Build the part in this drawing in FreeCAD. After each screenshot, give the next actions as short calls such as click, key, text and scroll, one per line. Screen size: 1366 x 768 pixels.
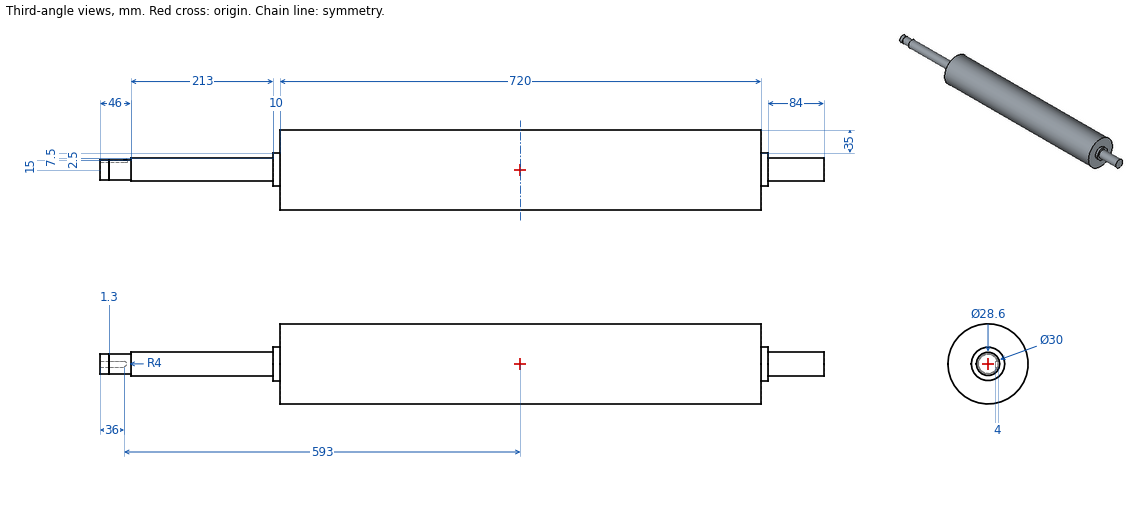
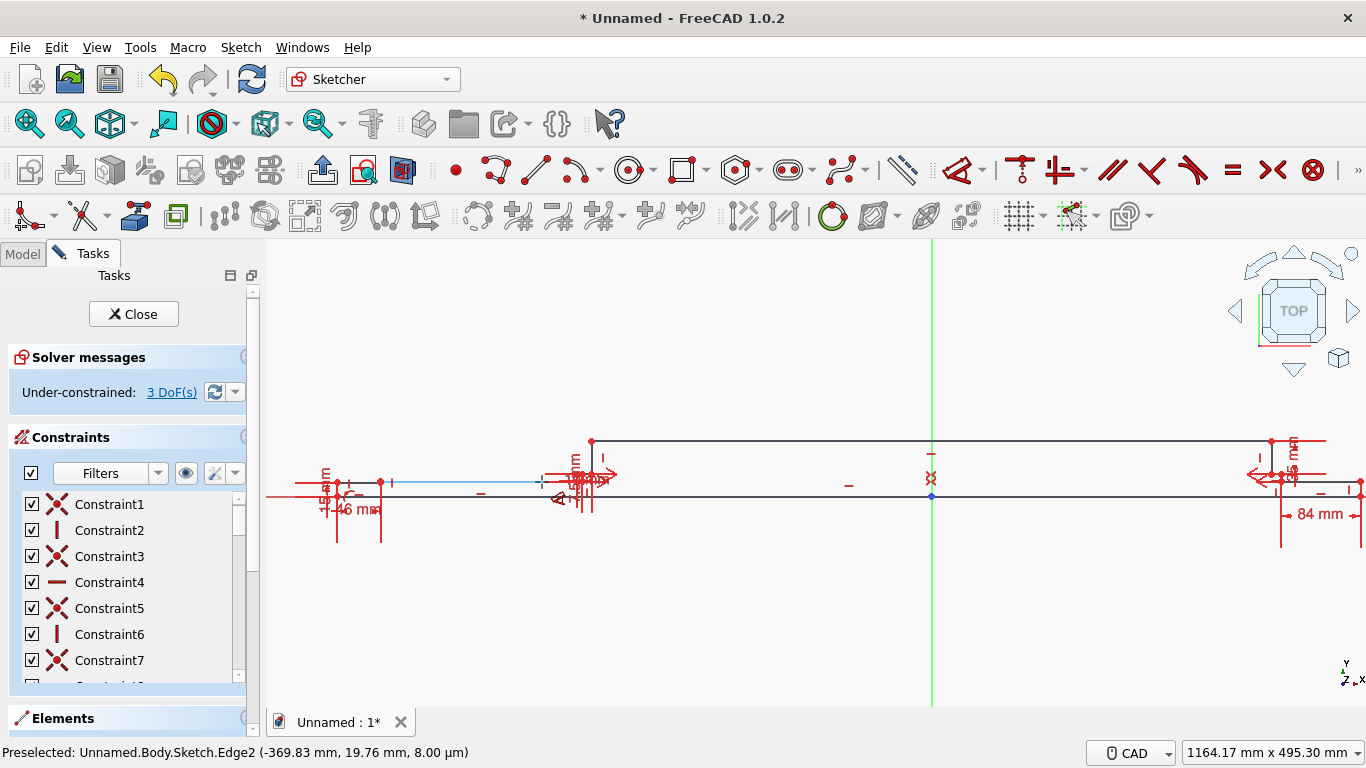
click(542, 481)
click(482, 515)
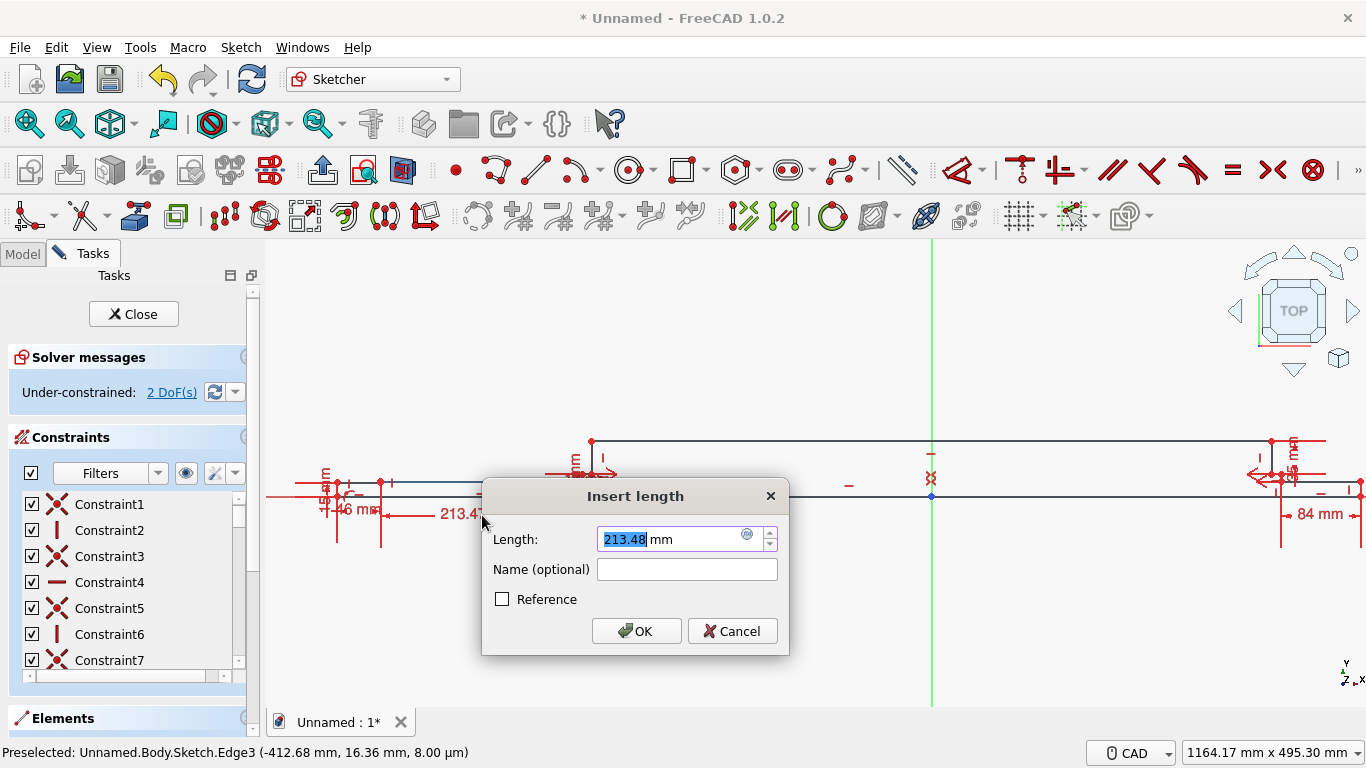
text(213)
key(Return)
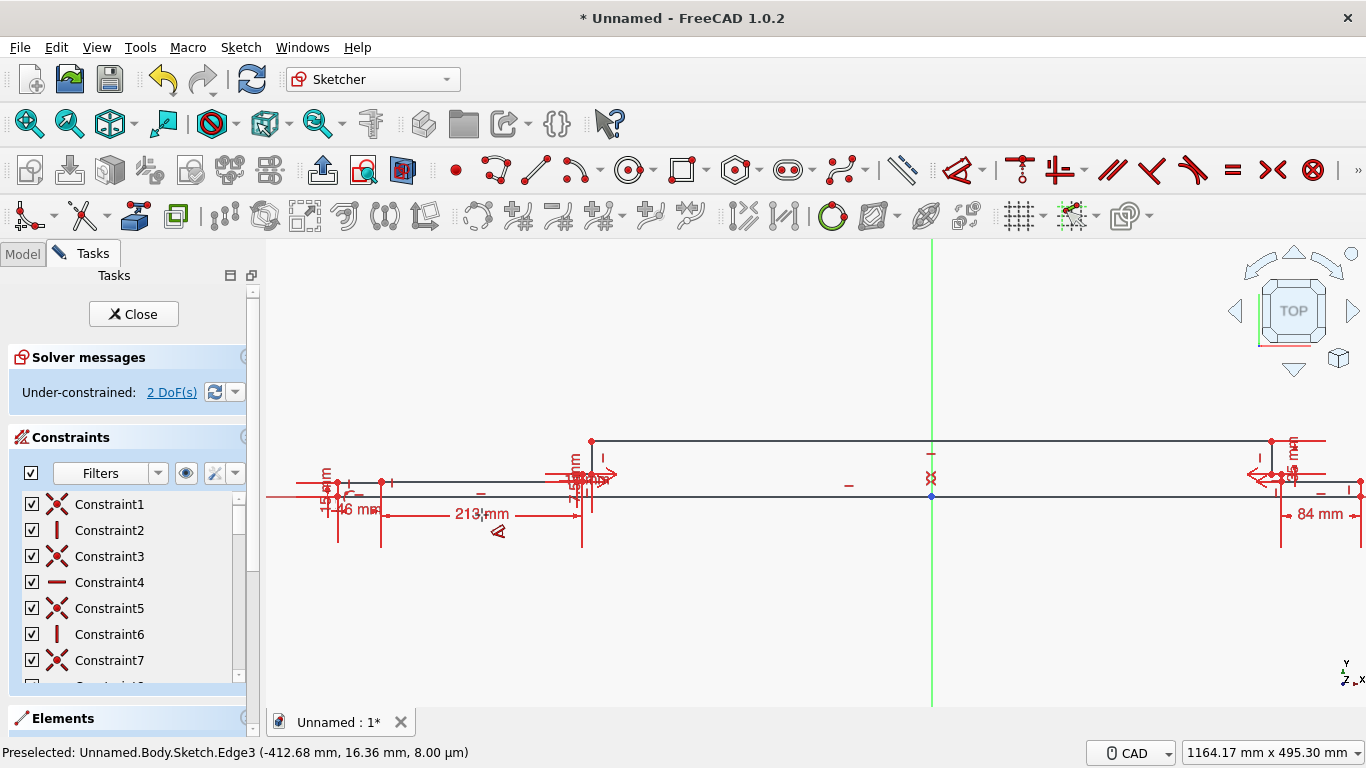
scroll(381, 482, up, 15)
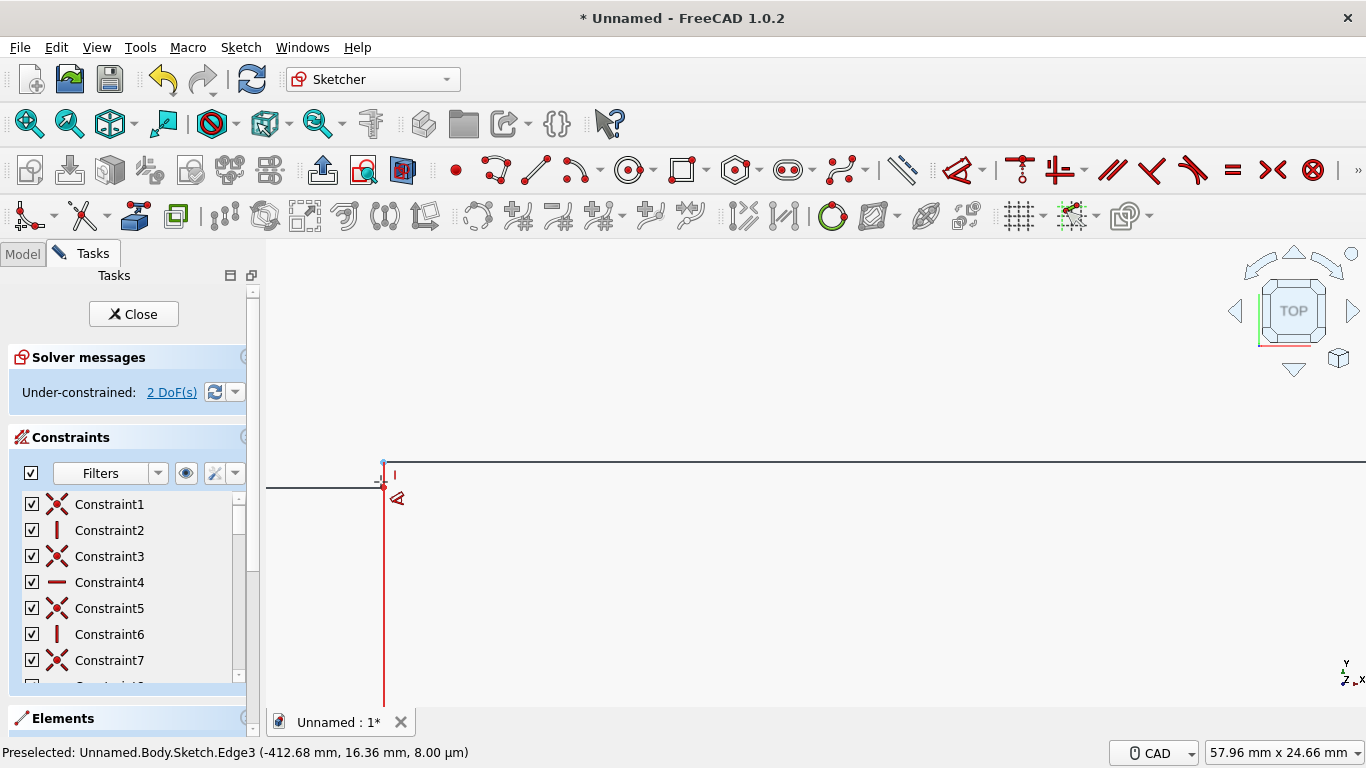
click(384, 475)
click(350, 469)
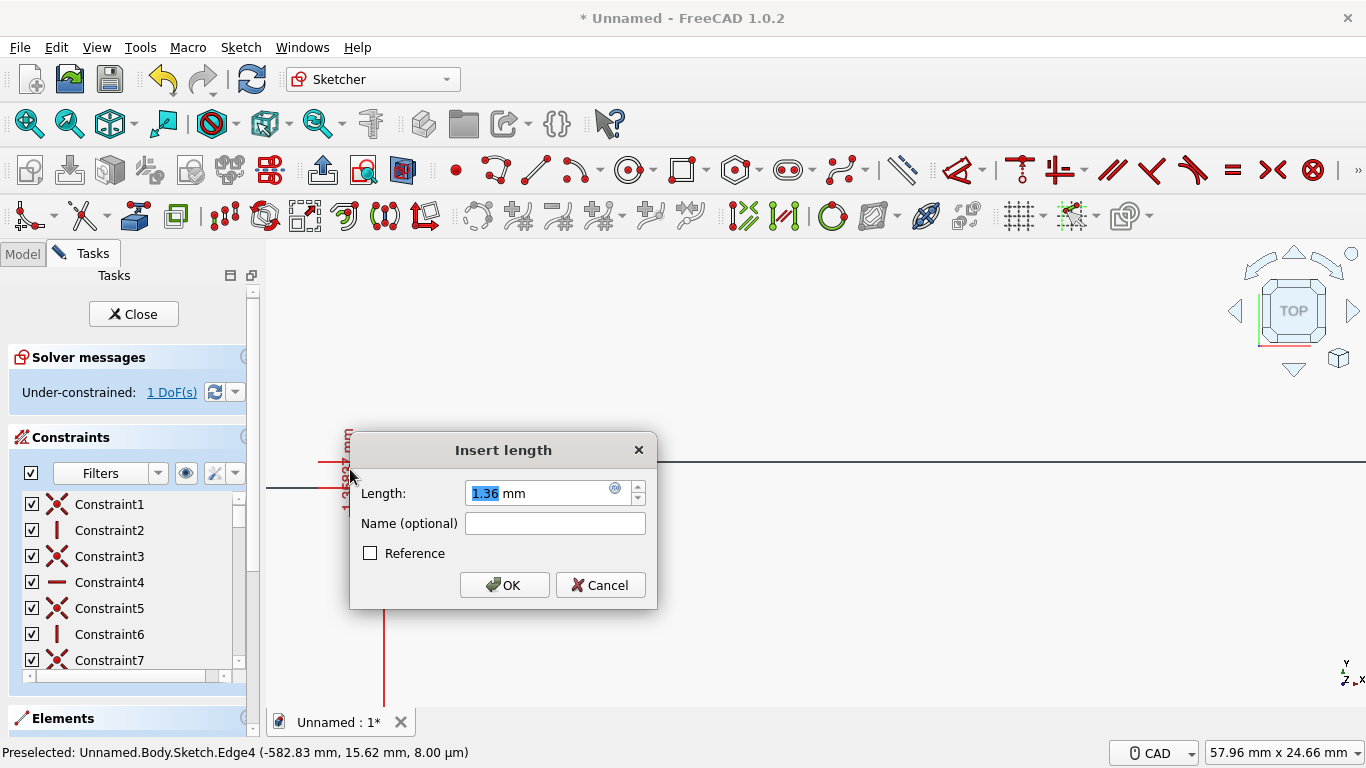
text(2.5)
key(Return)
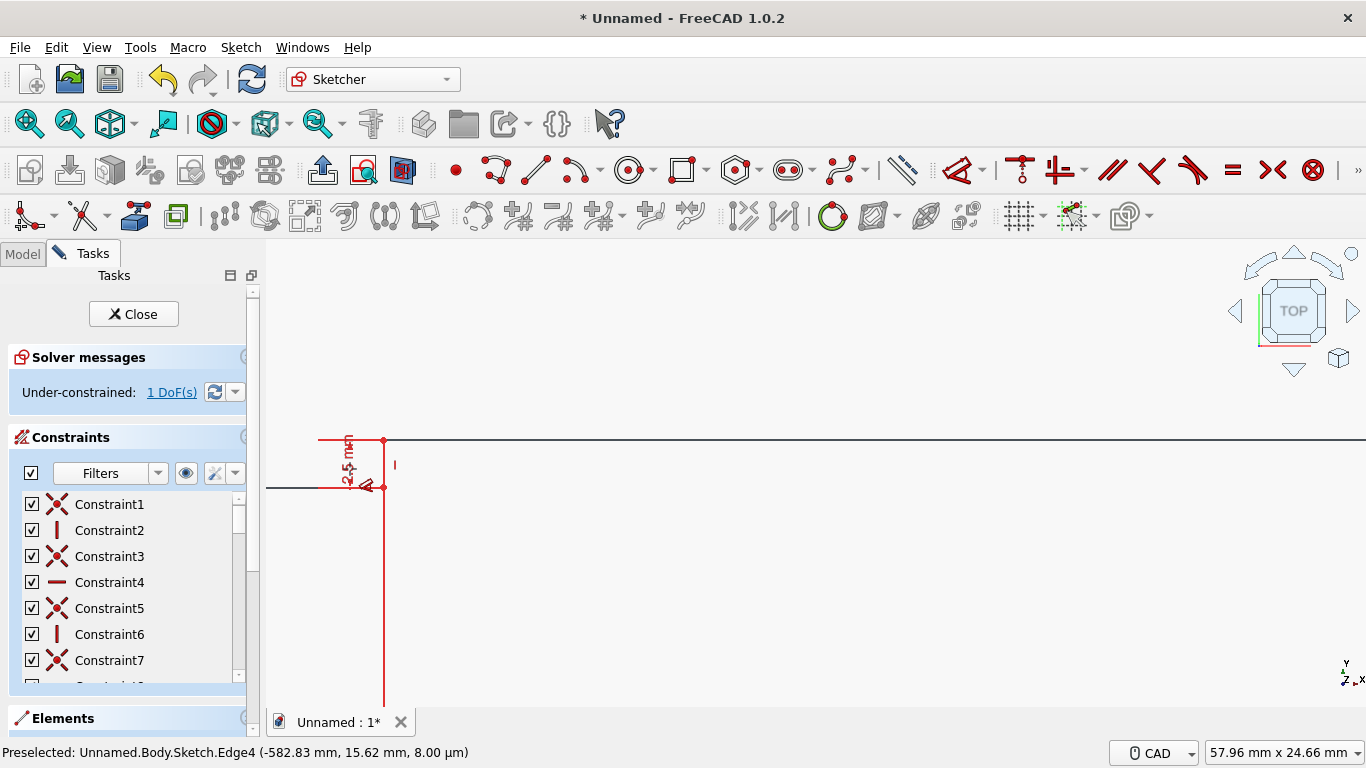
scroll(363, 484, down, 16)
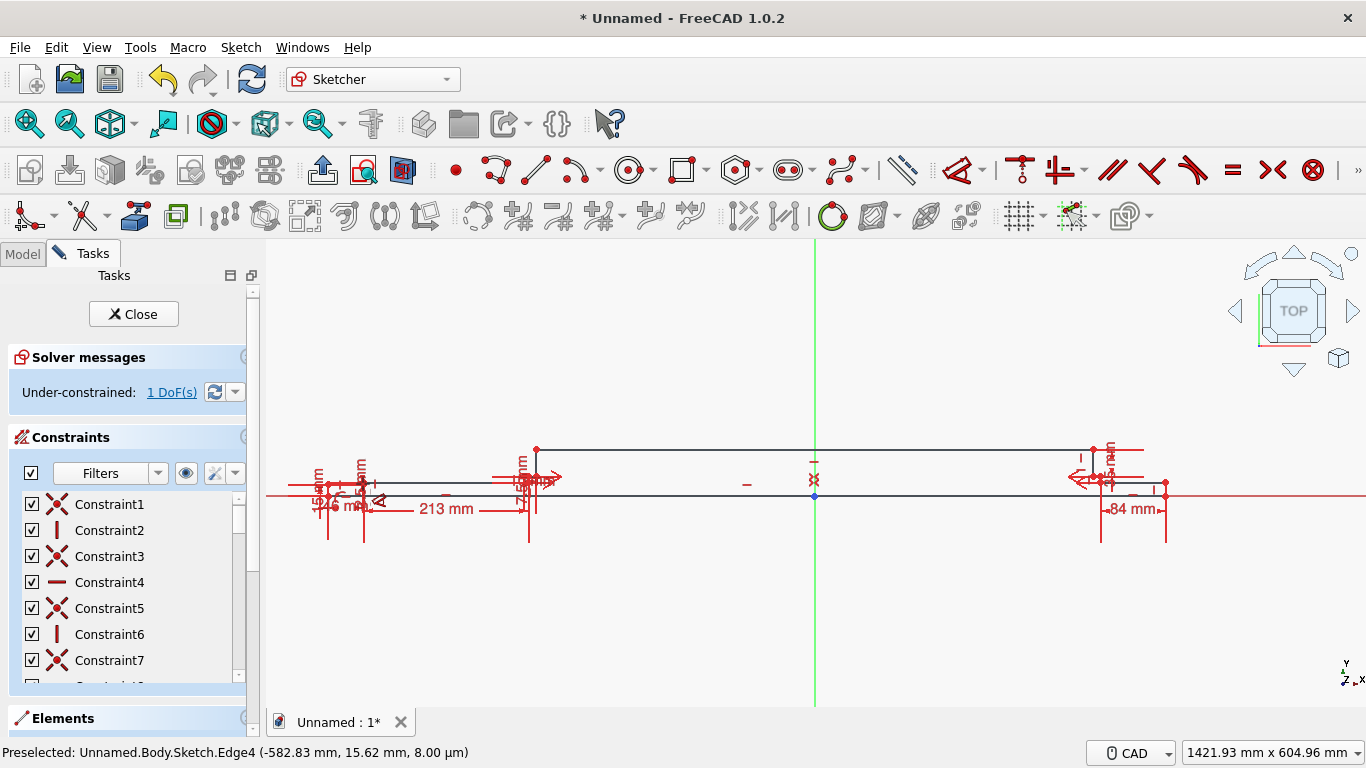
click(926, 450)
click(687, 416)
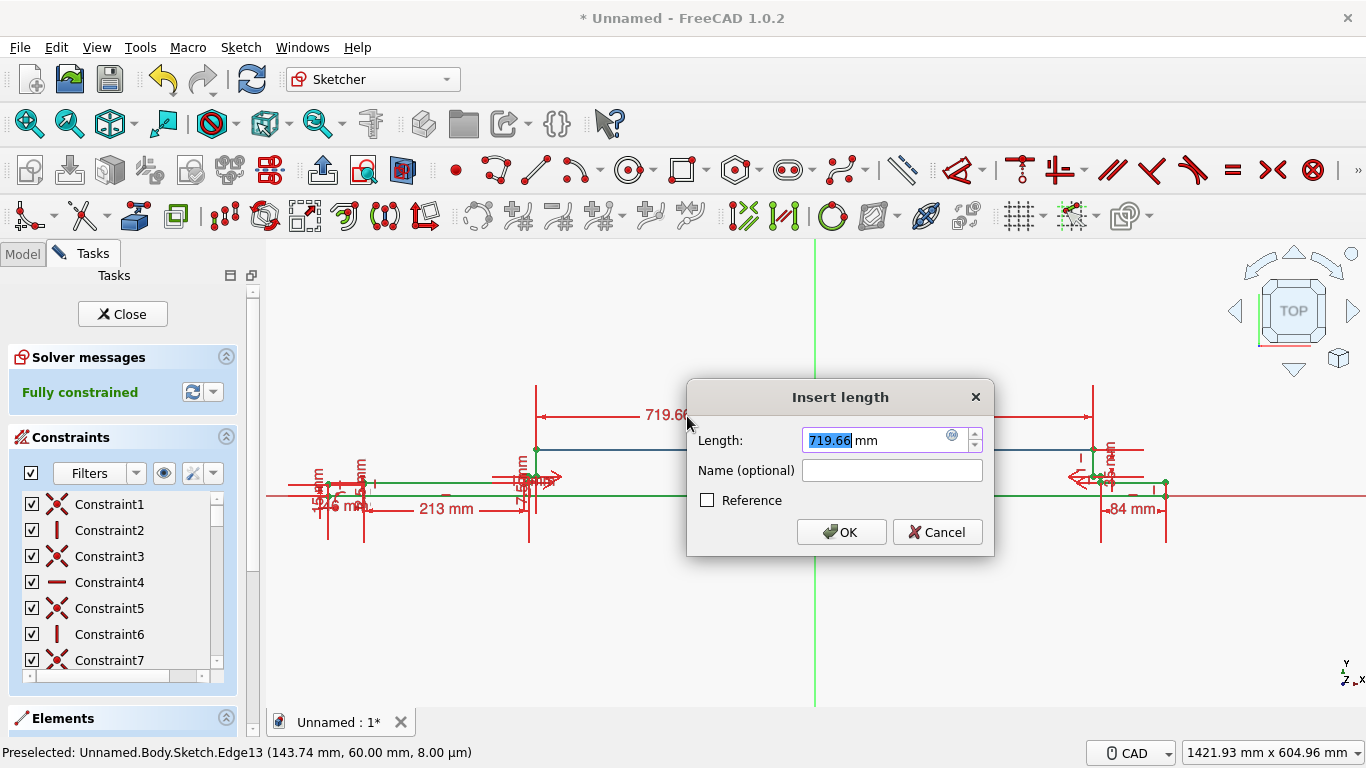
text(720)
key(Return)
key(Escape)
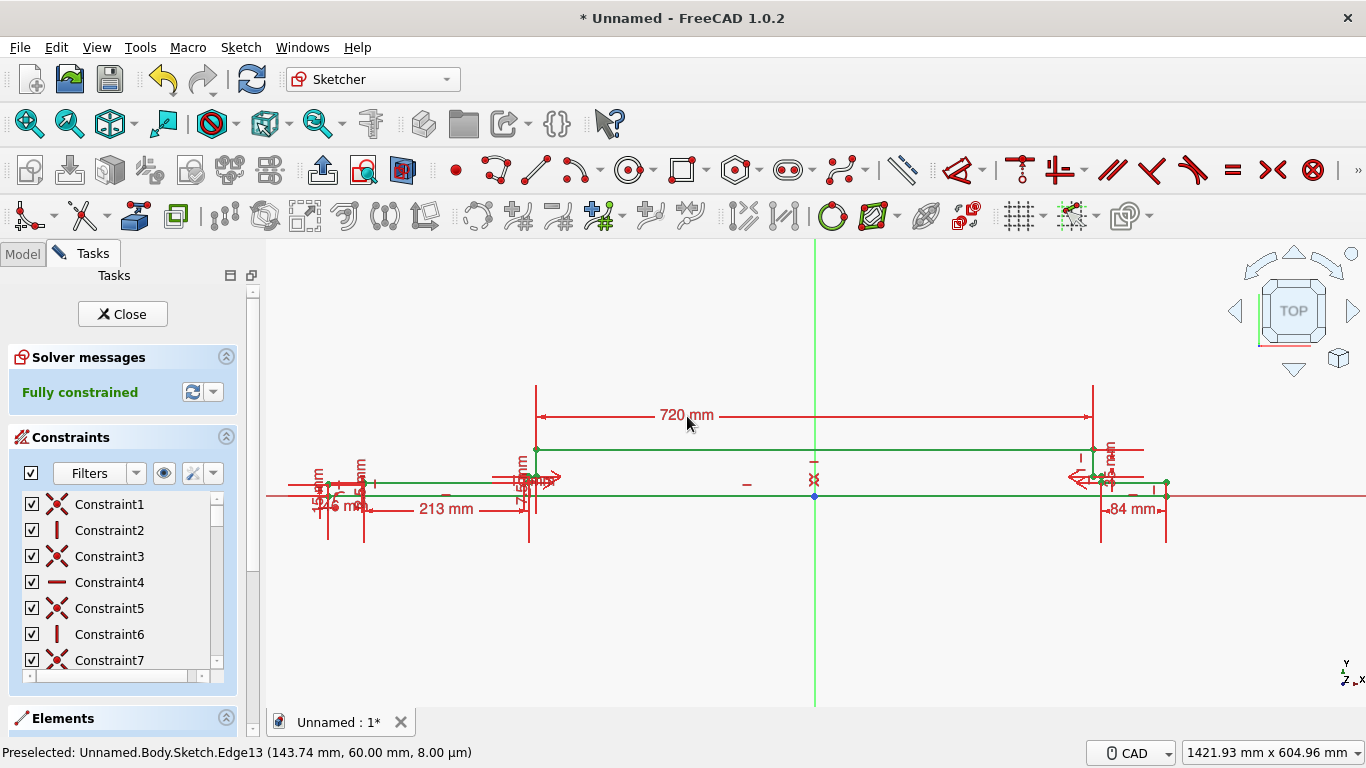
click(123, 314)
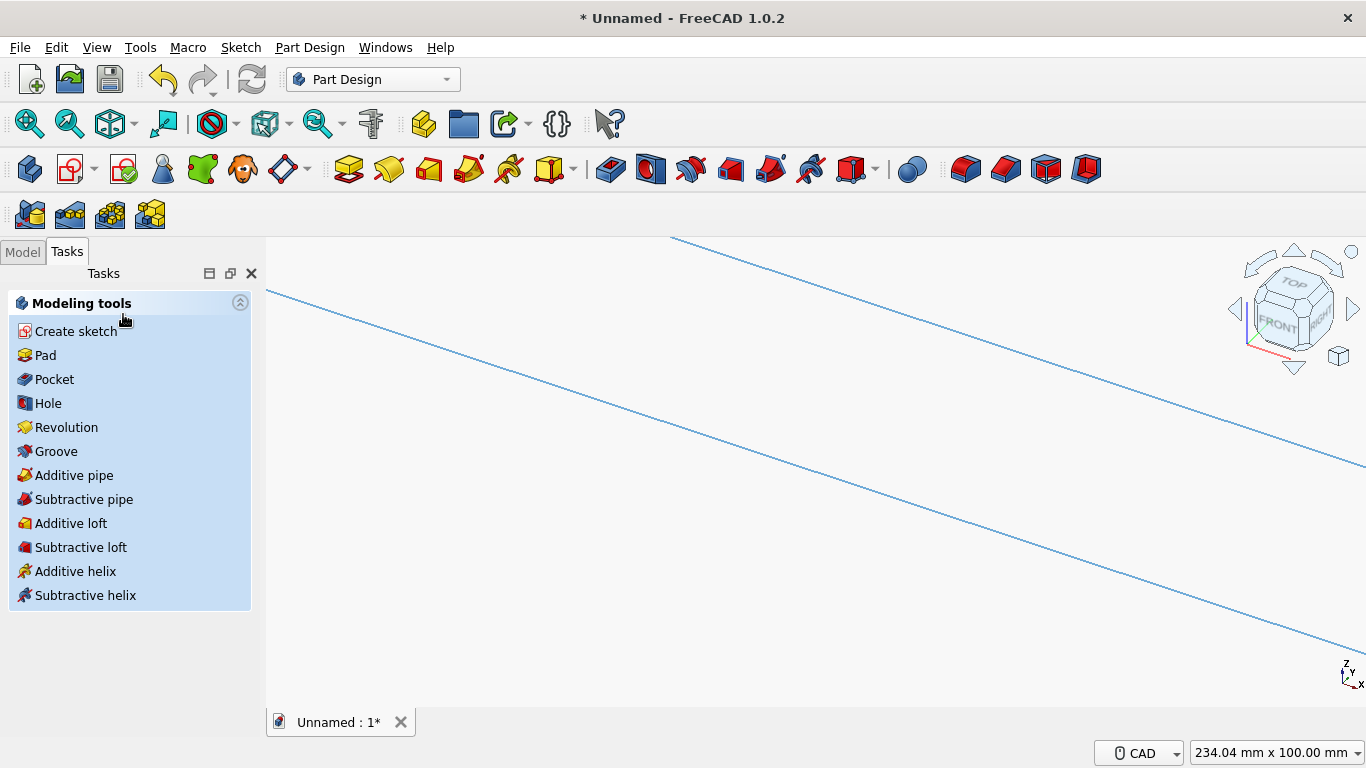
click(390, 170)